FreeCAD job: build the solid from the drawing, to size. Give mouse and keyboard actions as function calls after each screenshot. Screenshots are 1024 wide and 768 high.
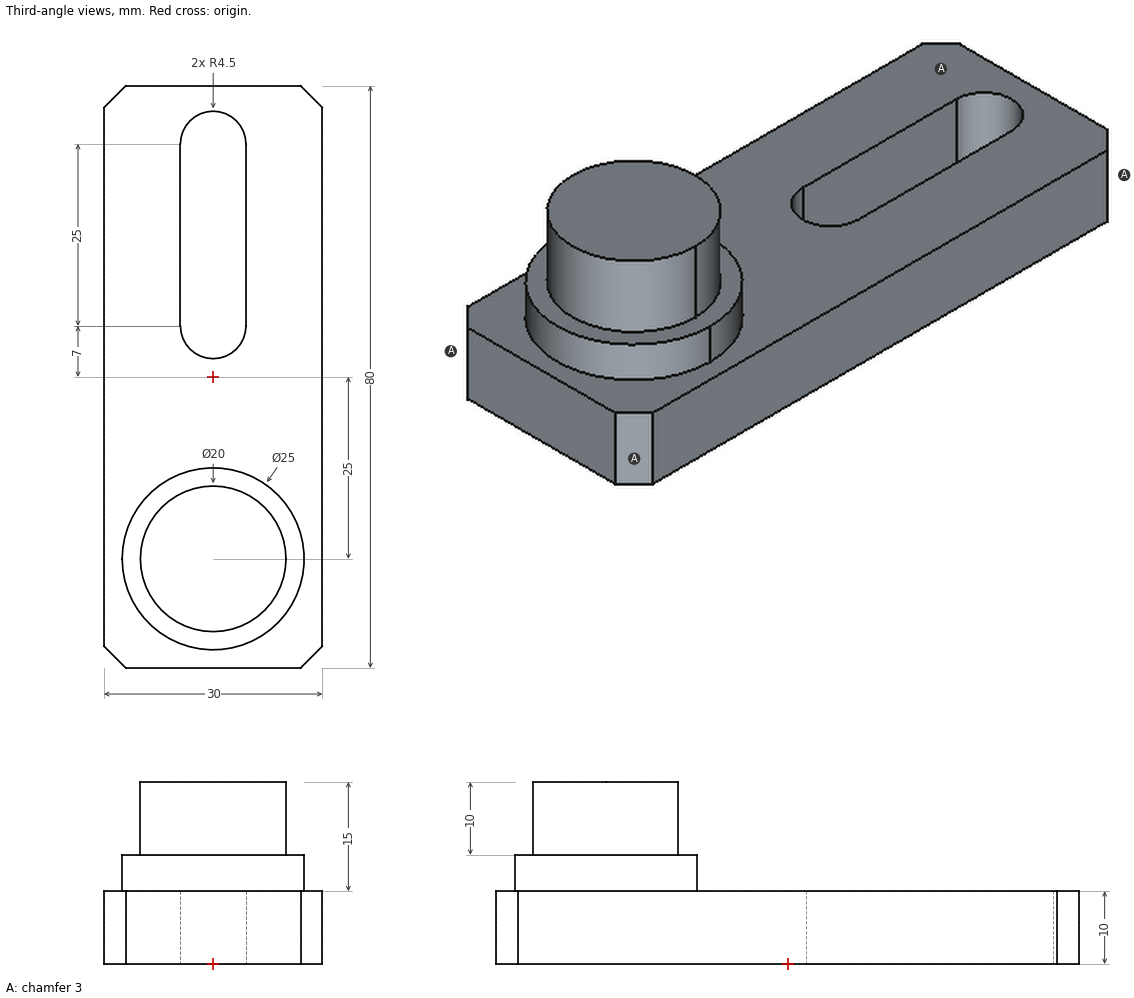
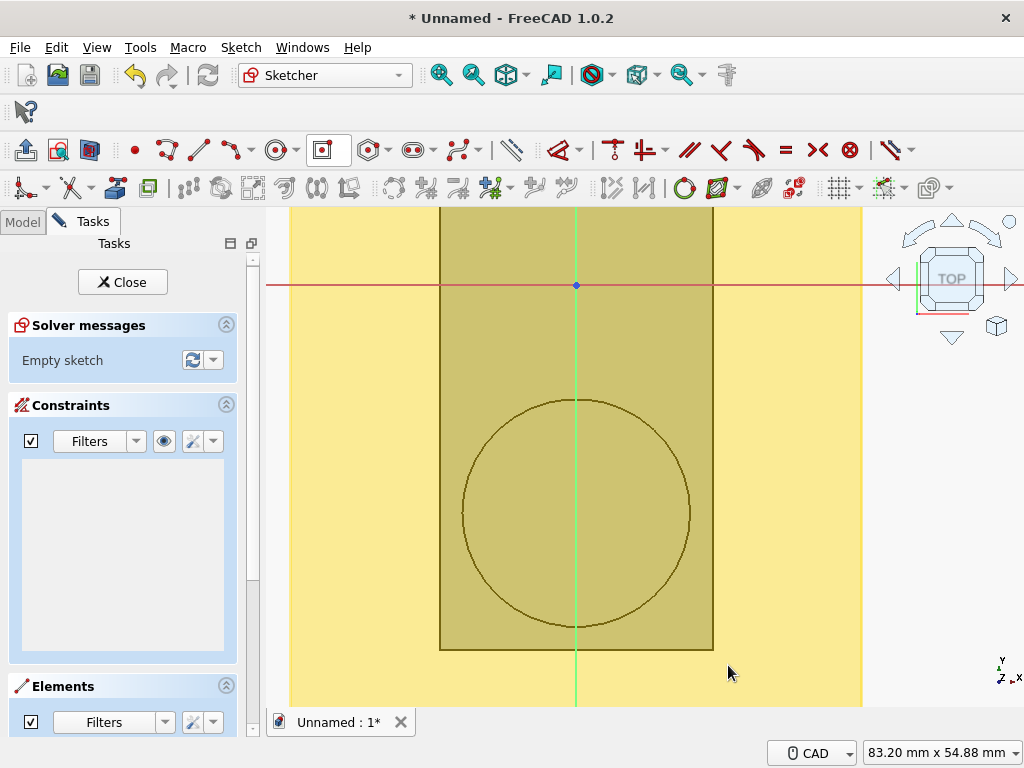
click(276, 150)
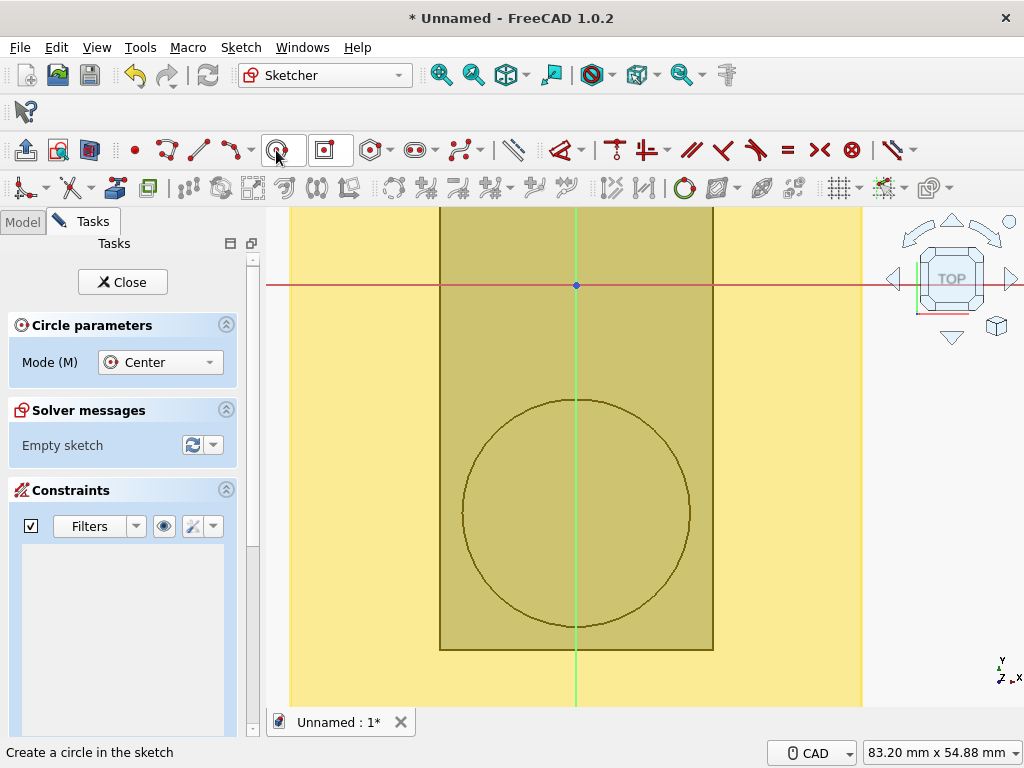
click(576, 513)
move(657, 432)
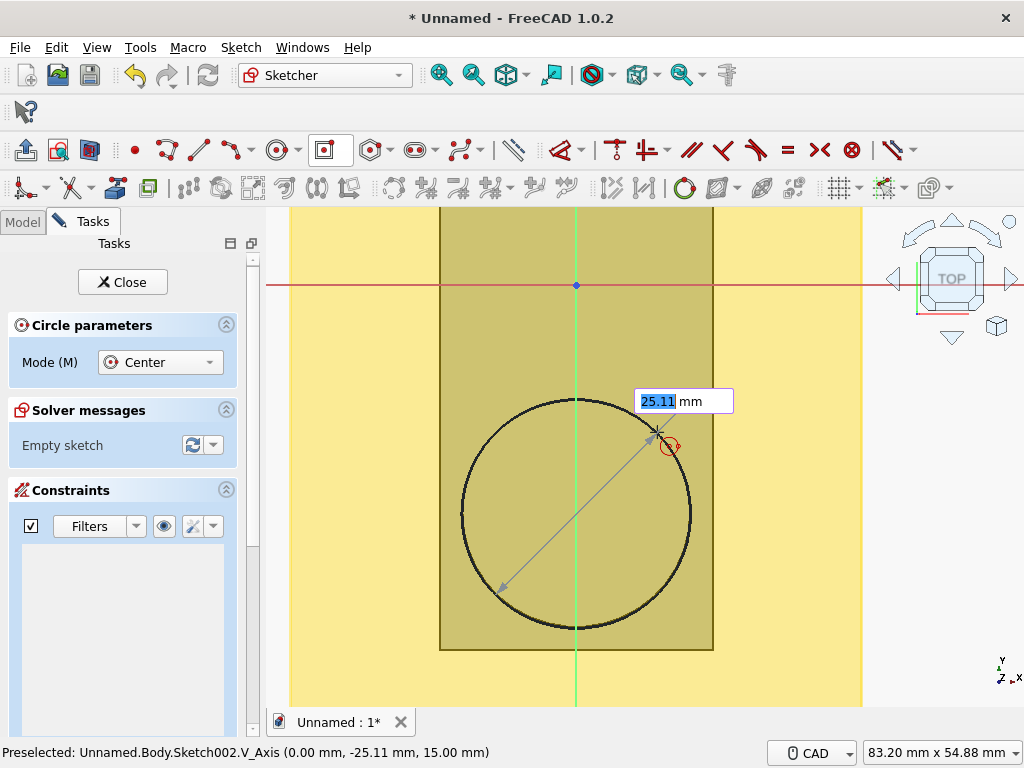
text(25)
key(Return)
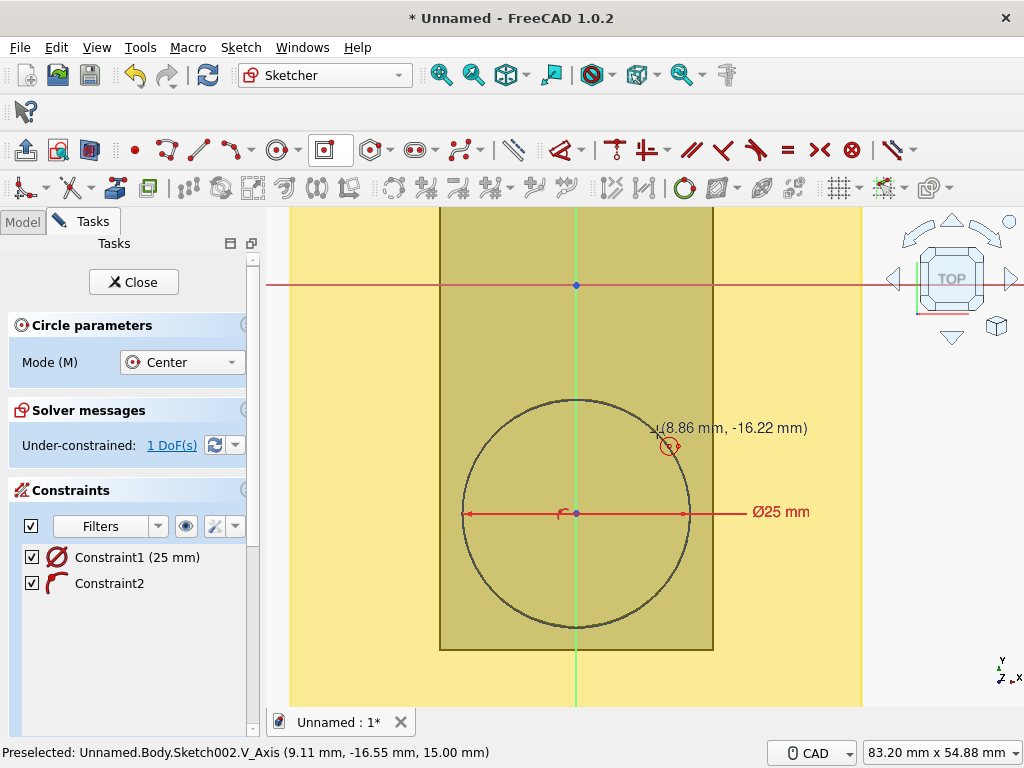
click(576, 514)
move(641, 449)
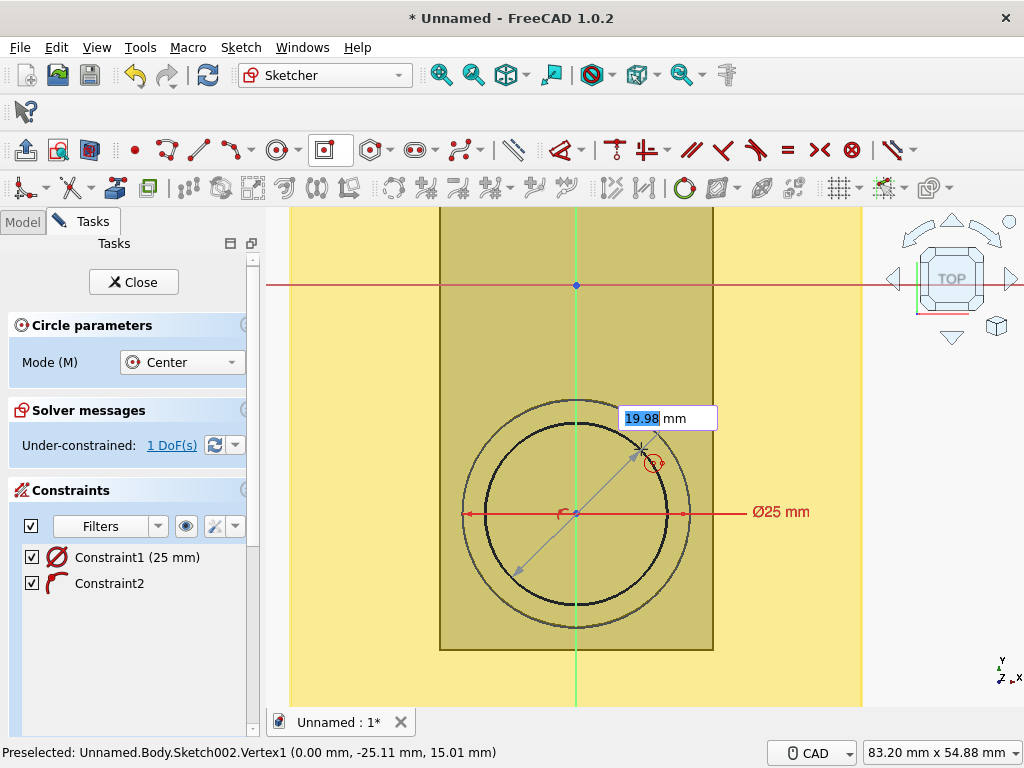
text(20)
key(Return)
key(Escape)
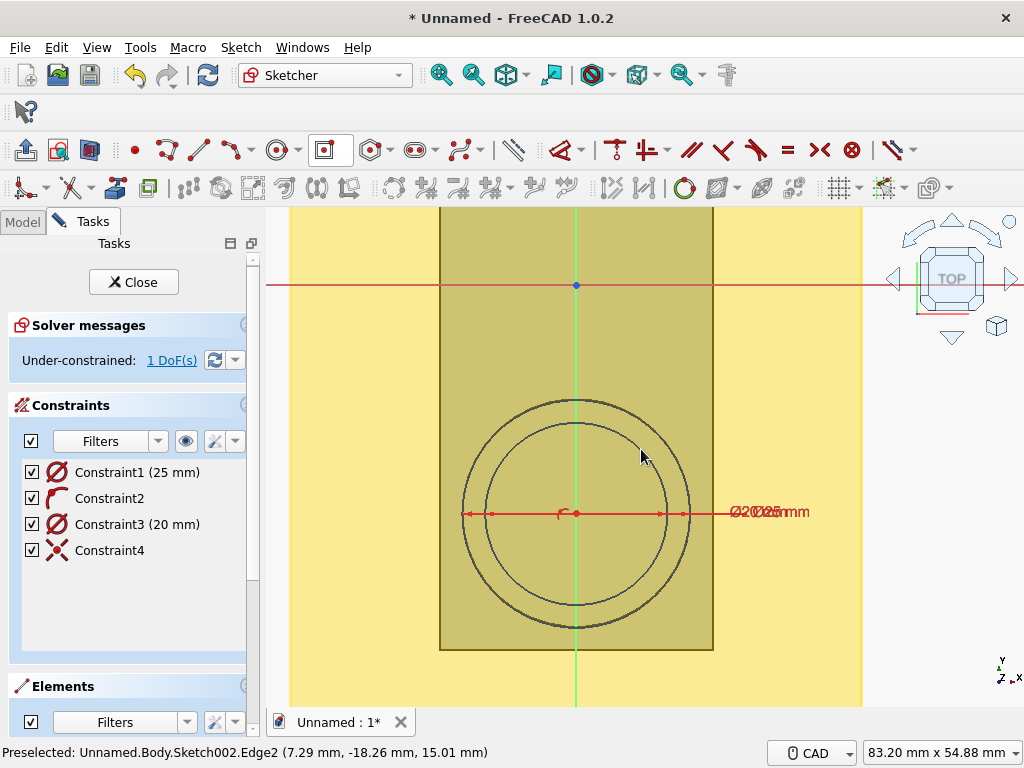
click(560, 150)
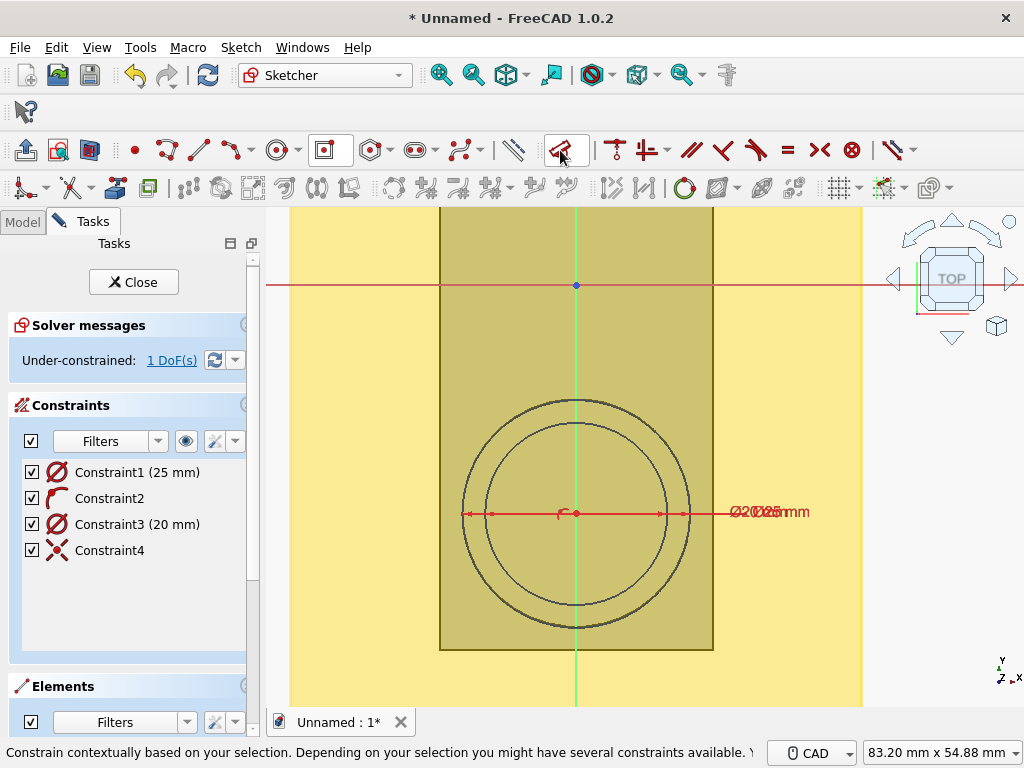
click(576, 514)
click(610, 347)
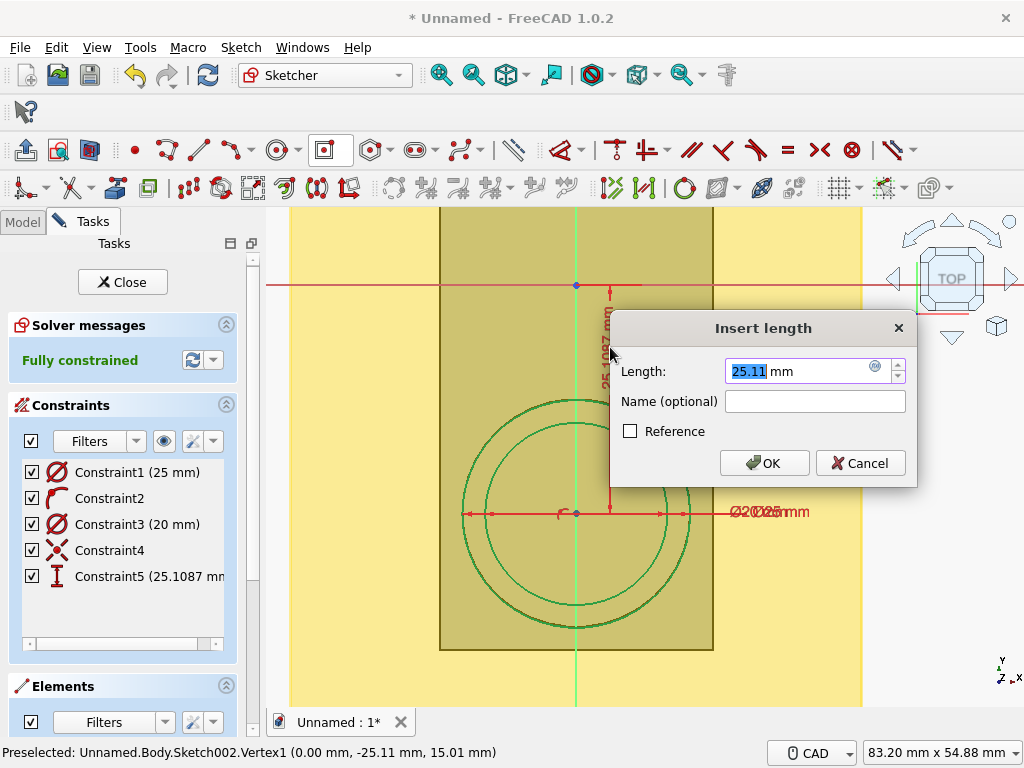
text(25)
key(Return)
key(Escape)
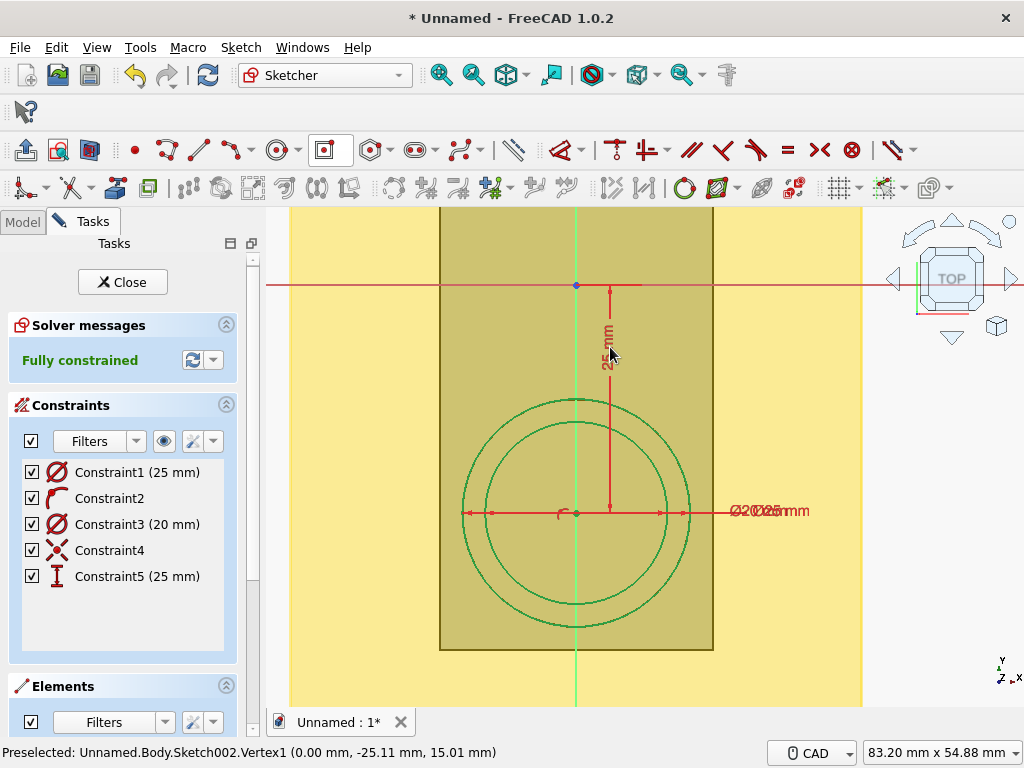
click(123, 282)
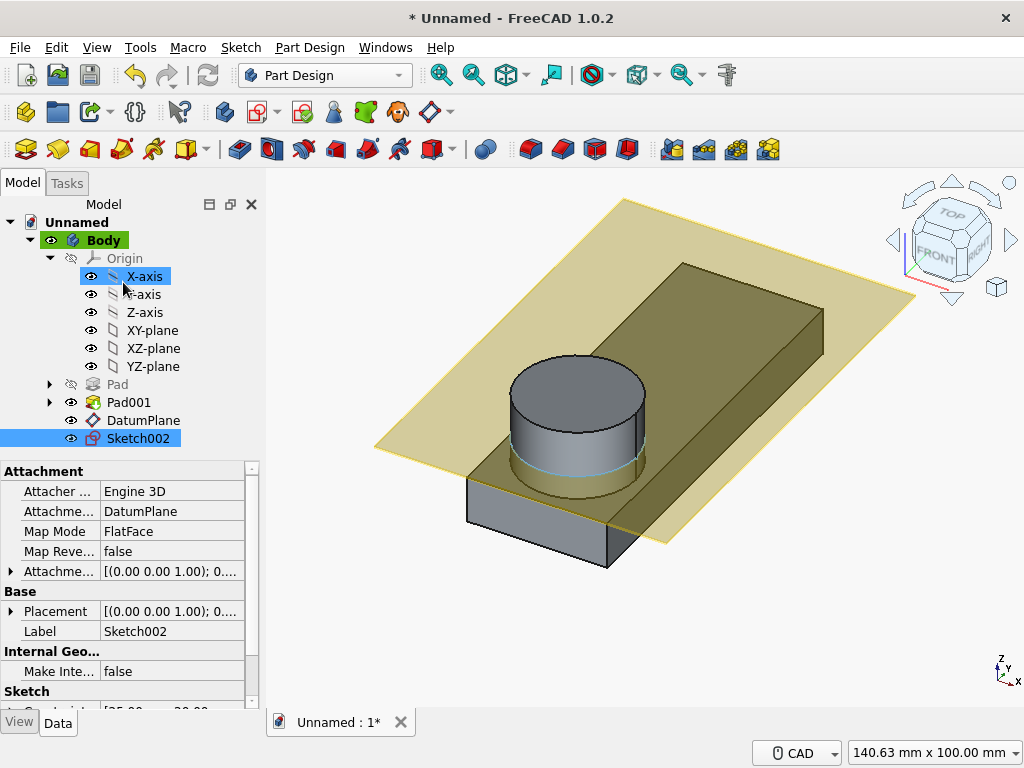
click(240, 150)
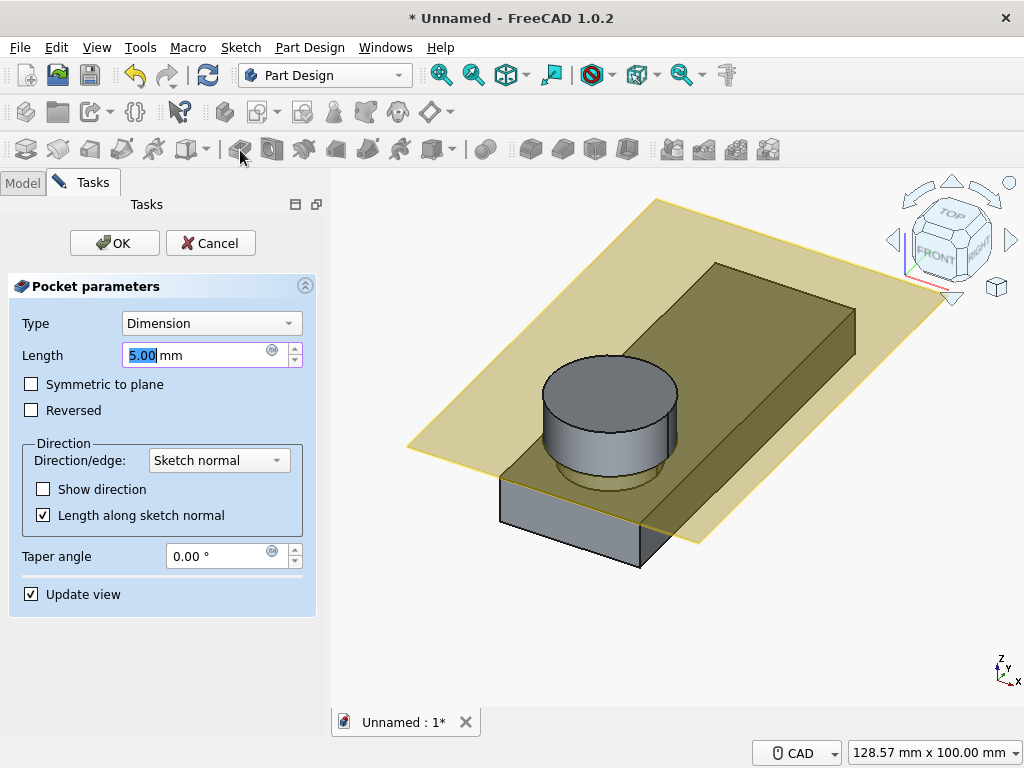
text(10)
key(Tab)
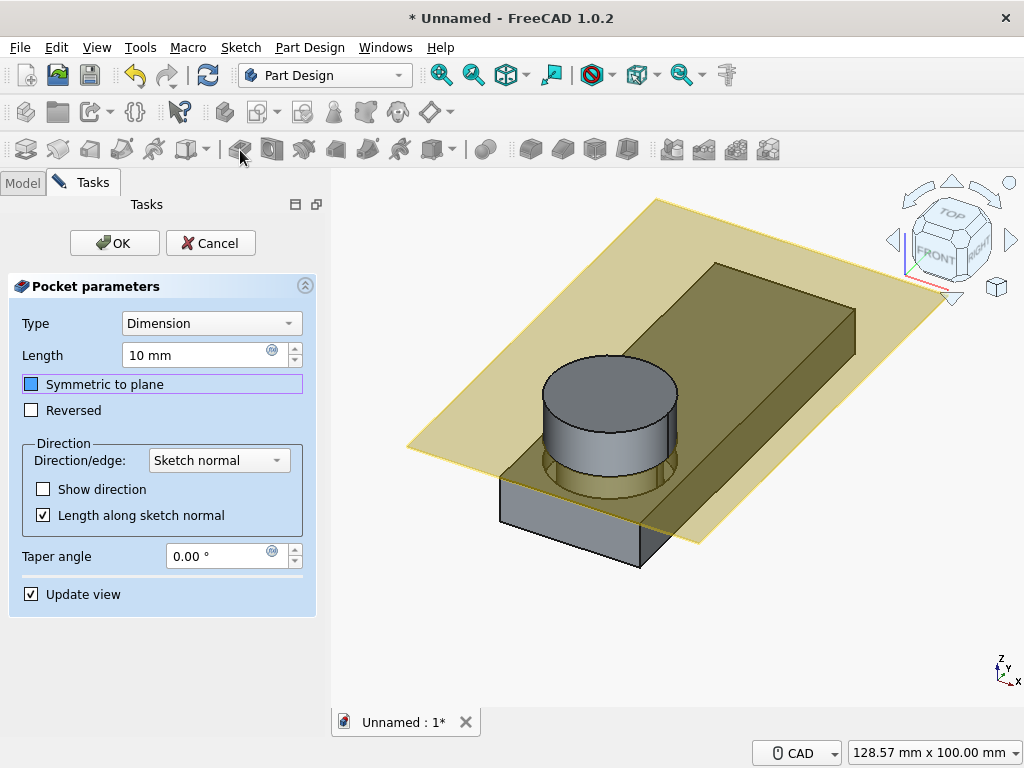
click(30, 410)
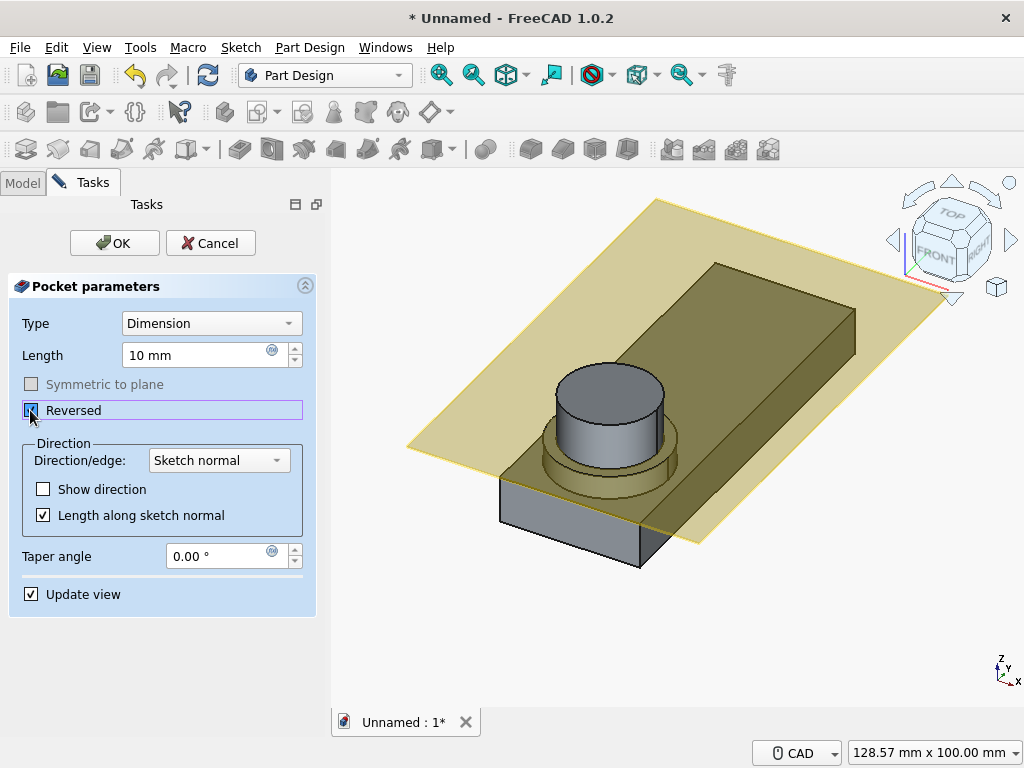
click(115, 243)